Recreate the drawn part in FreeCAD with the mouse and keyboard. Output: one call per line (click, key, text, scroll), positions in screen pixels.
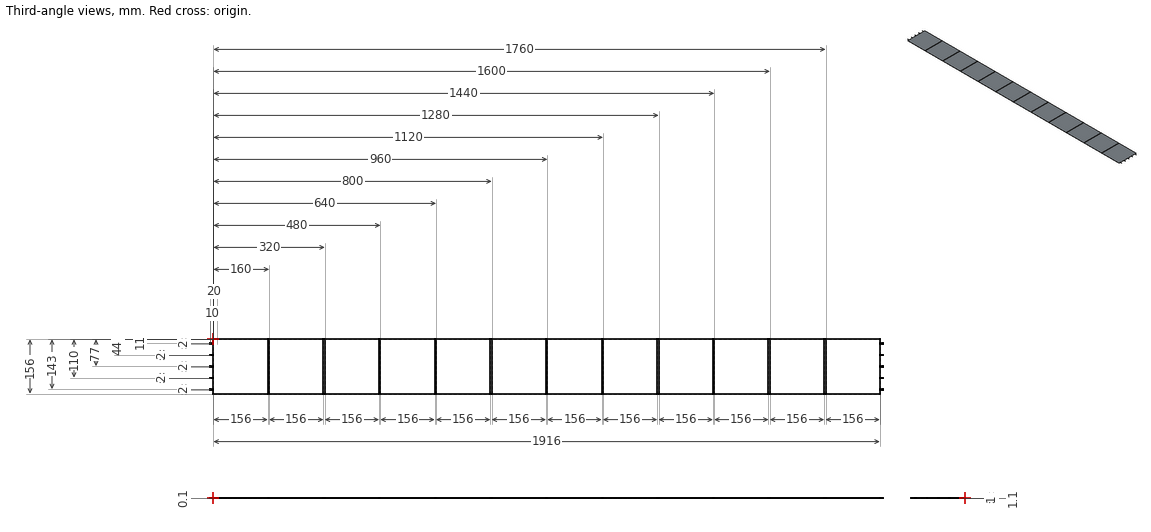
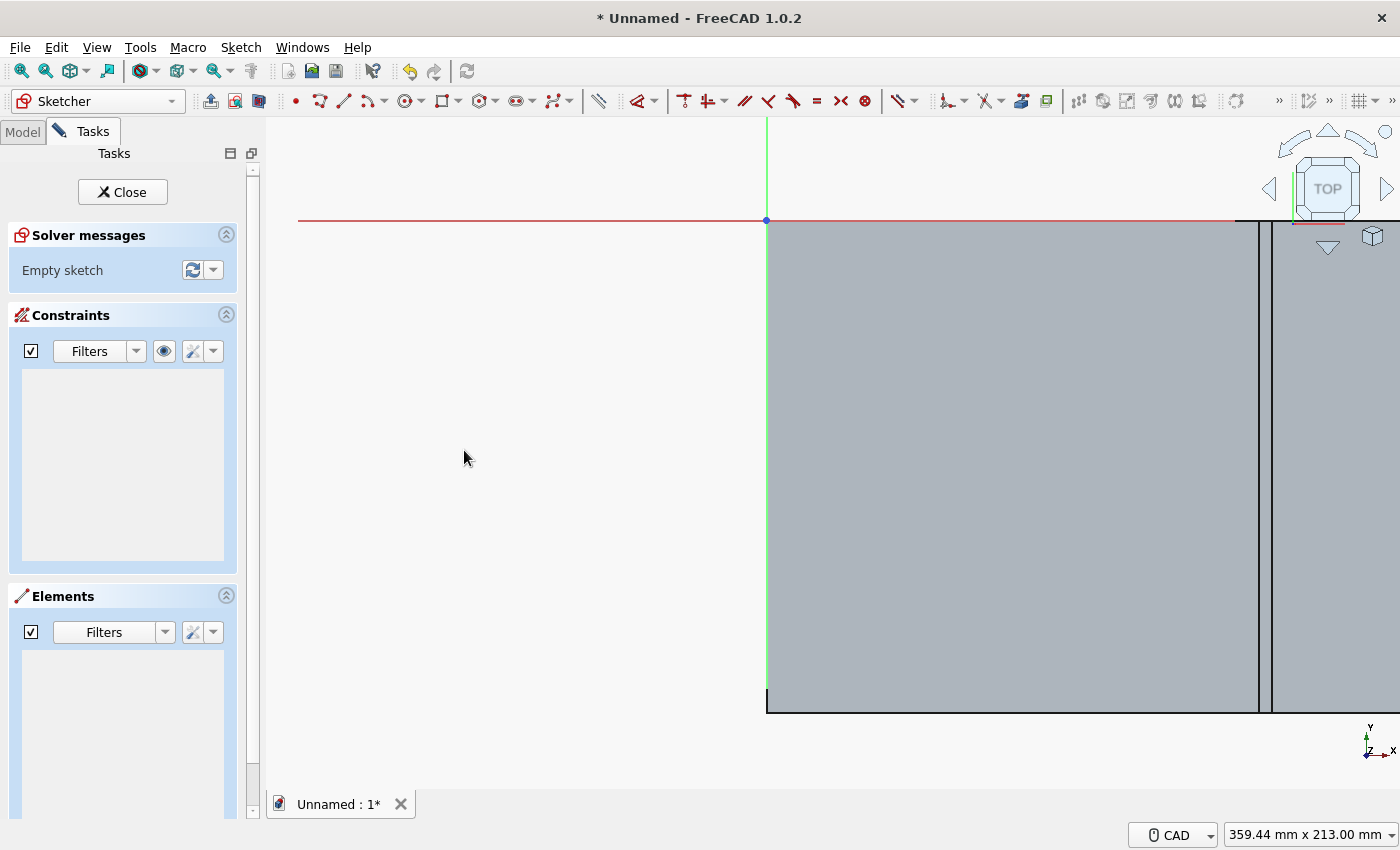
key(g)
key(r)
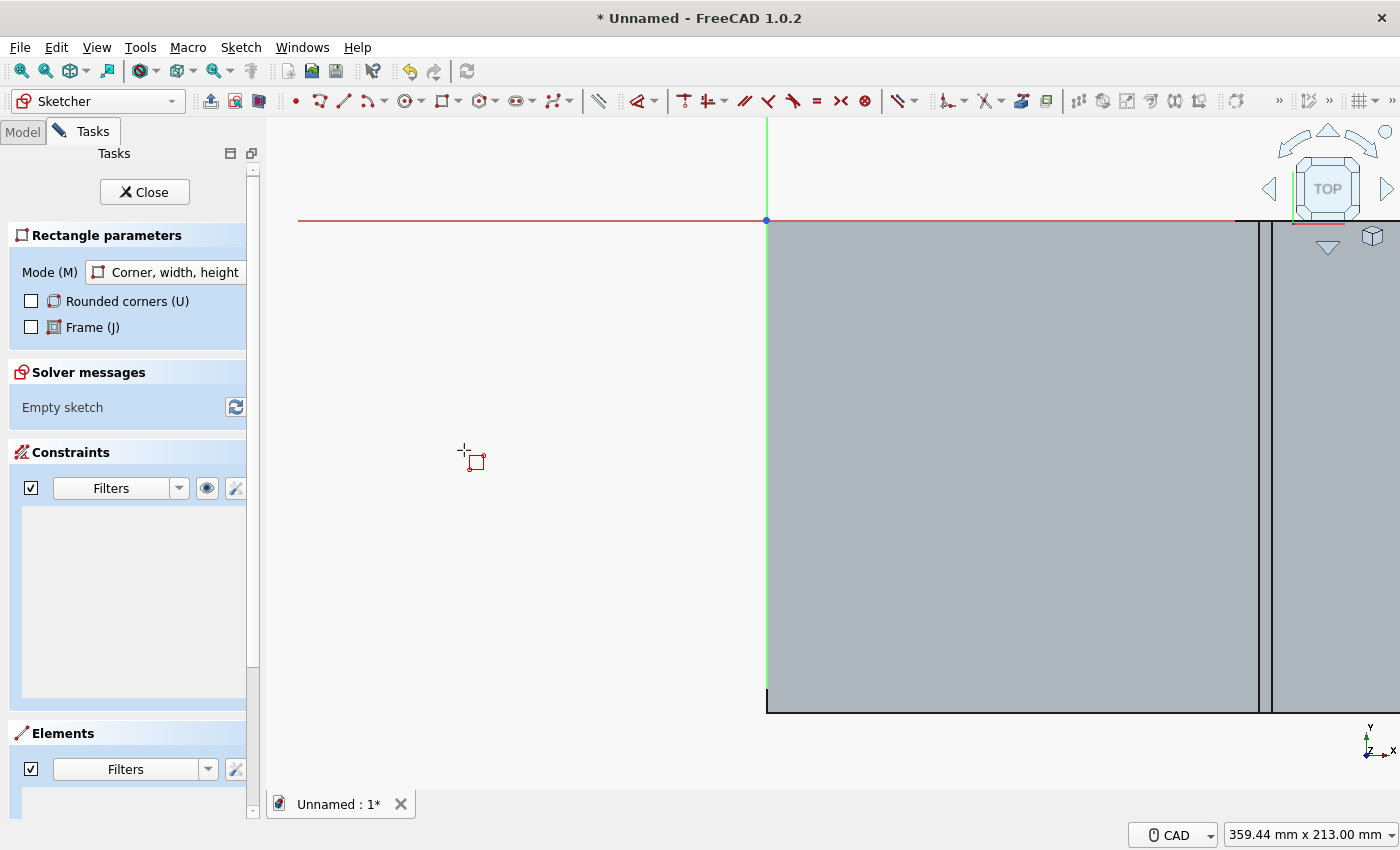
scroll(735, 255, up, 5)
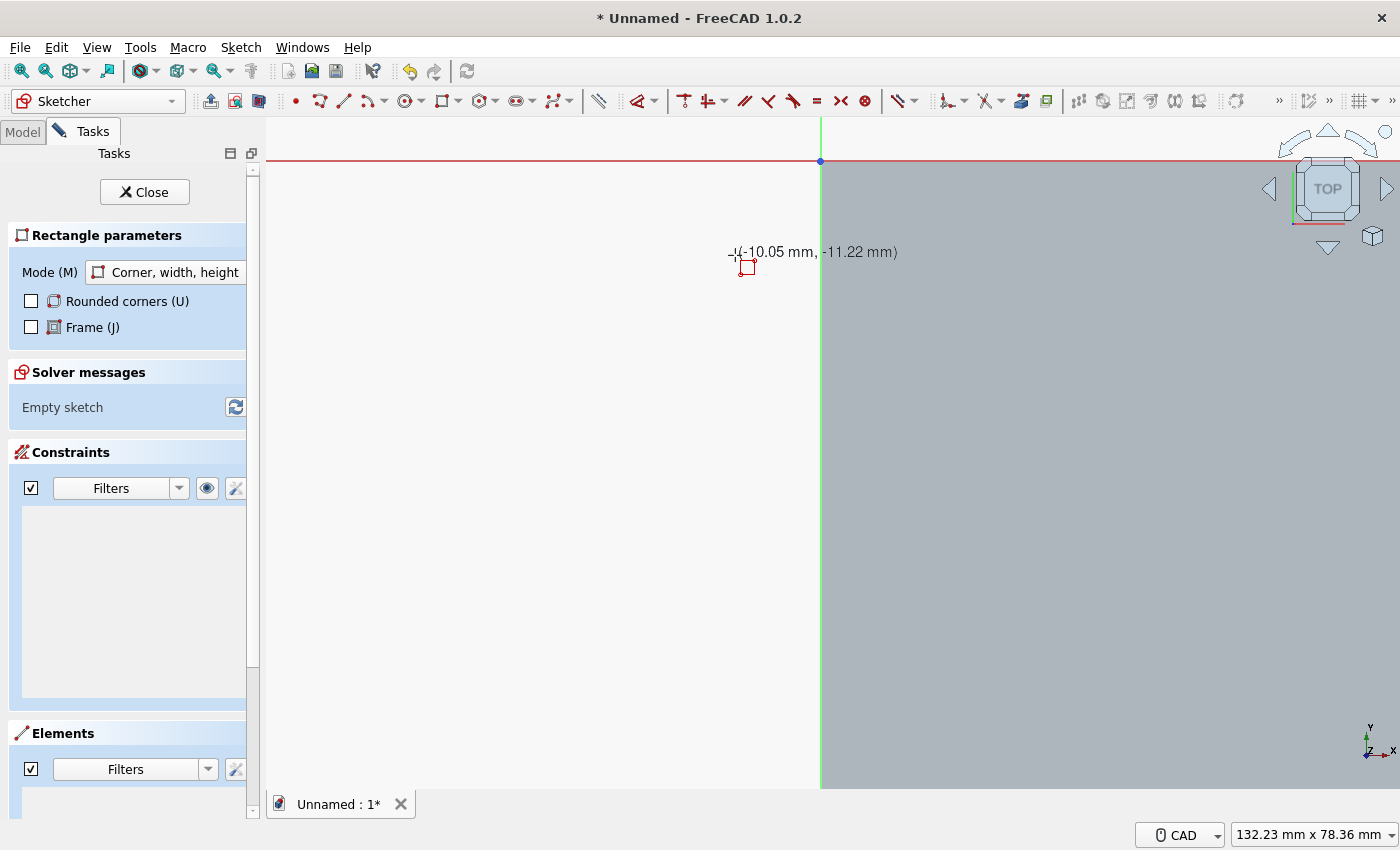
click(735, 255)
click(906, 273)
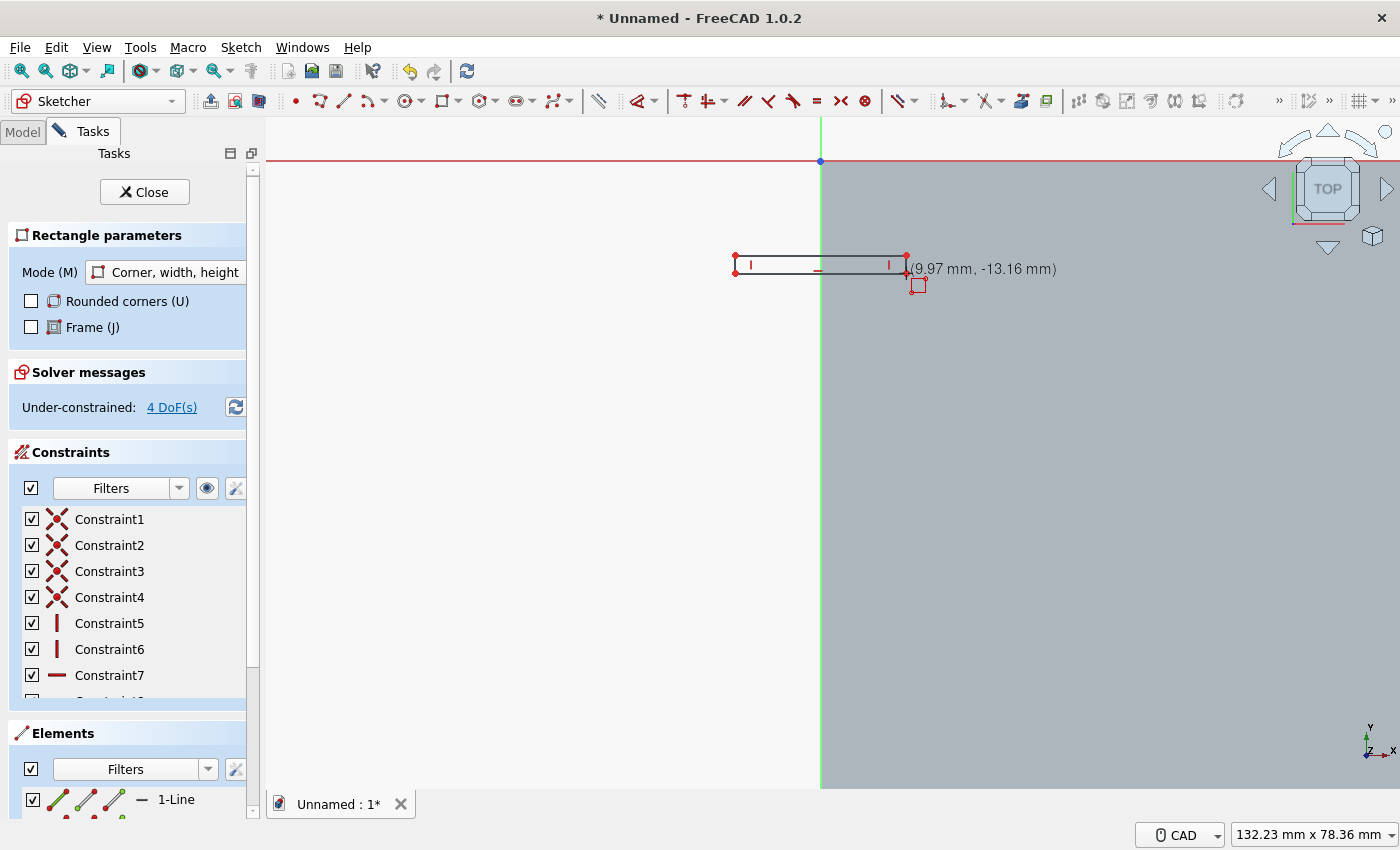
click(735, 538)
click(906, 556)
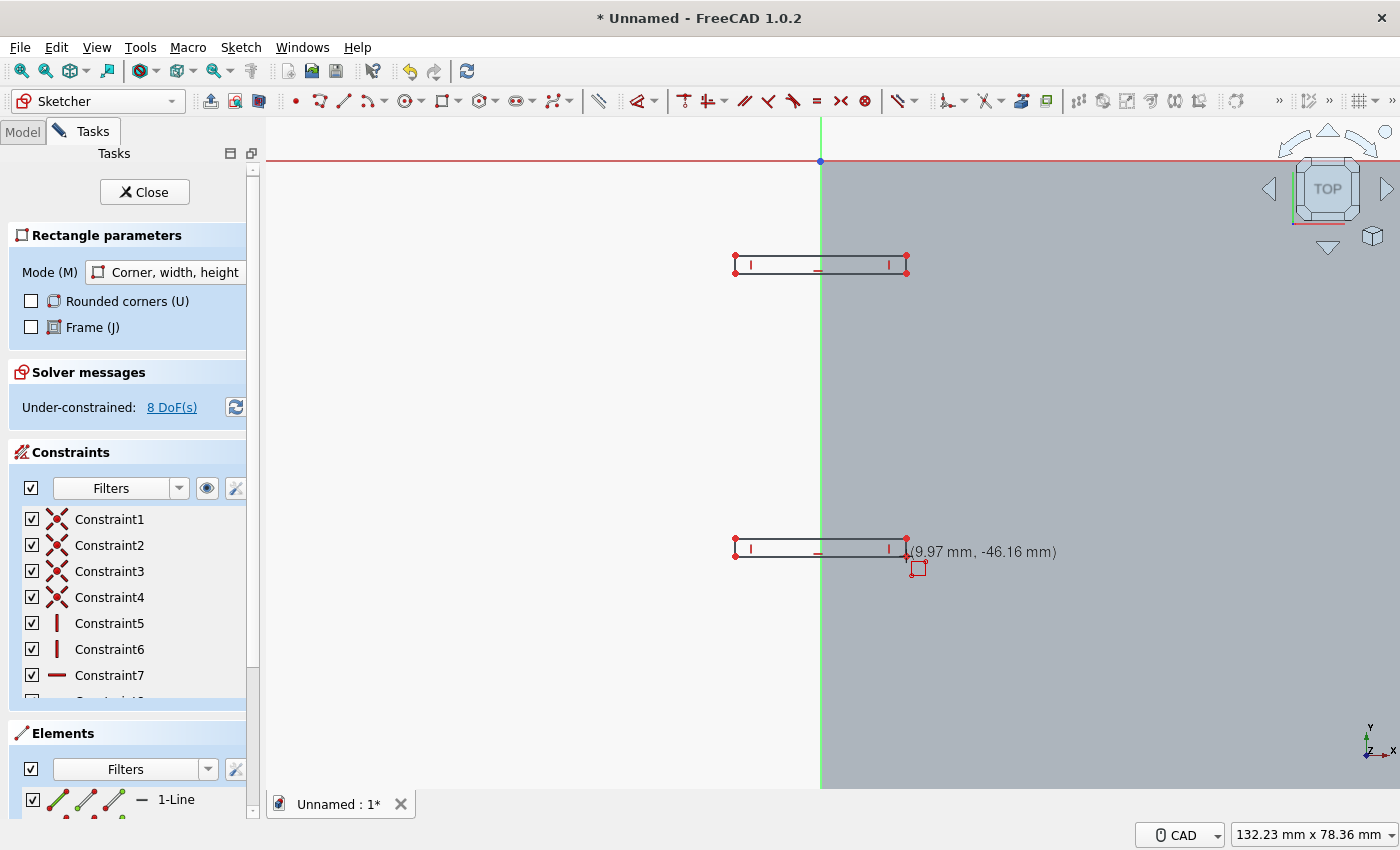
scroll(732, 261, down, 5)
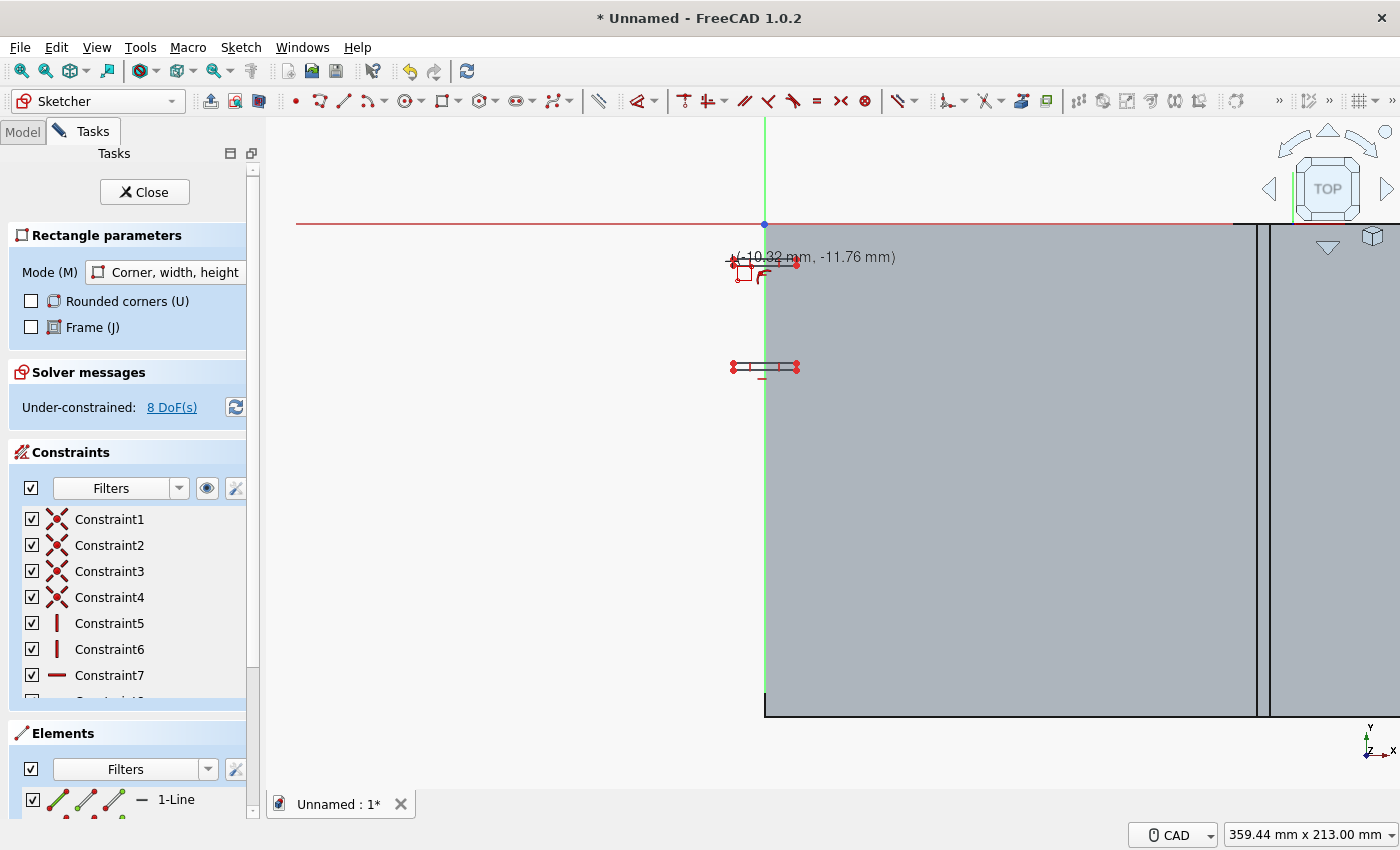
scroll(733, 467, up, 5)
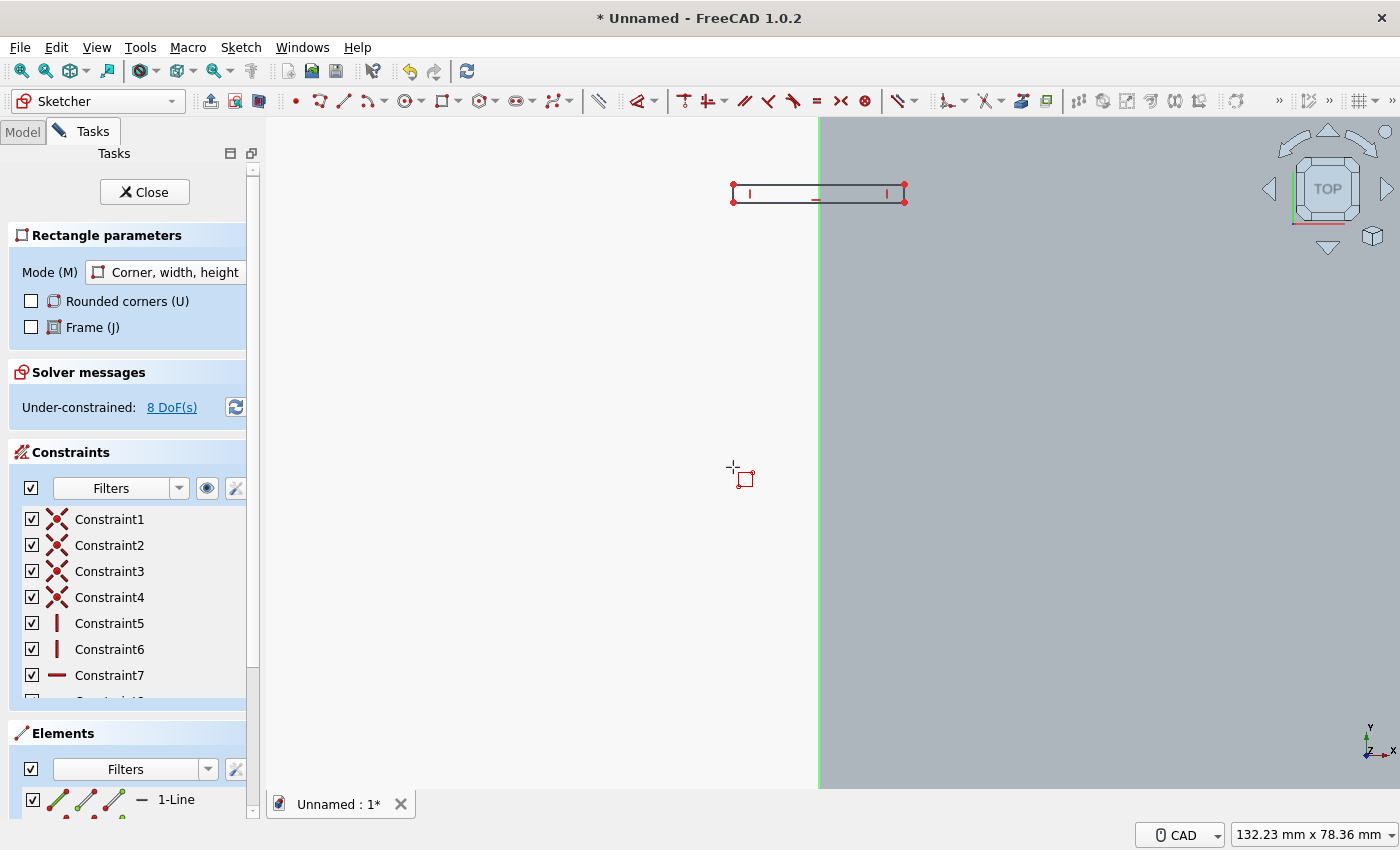
click(733, 467)
click(905, 484)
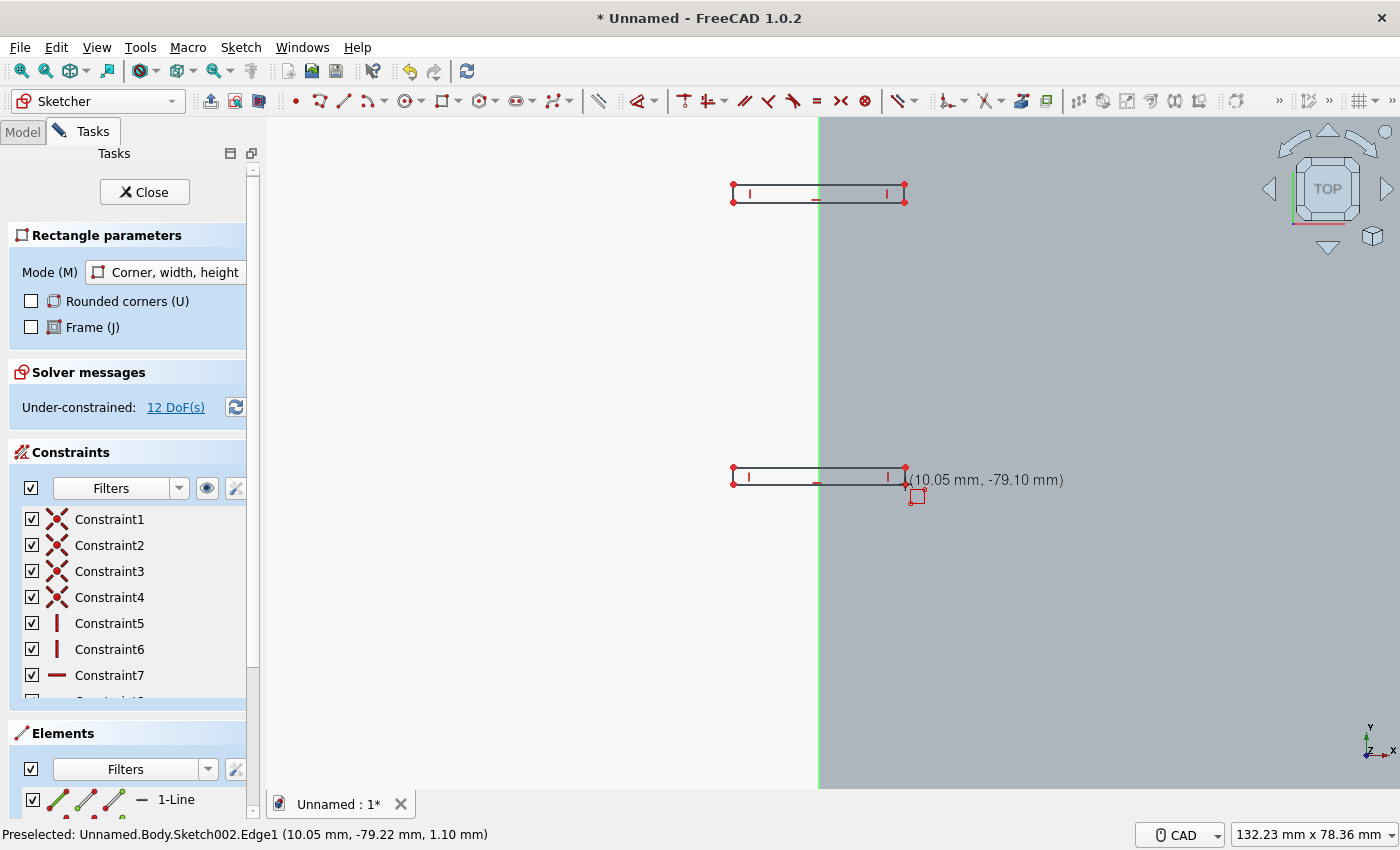
click(733, 750)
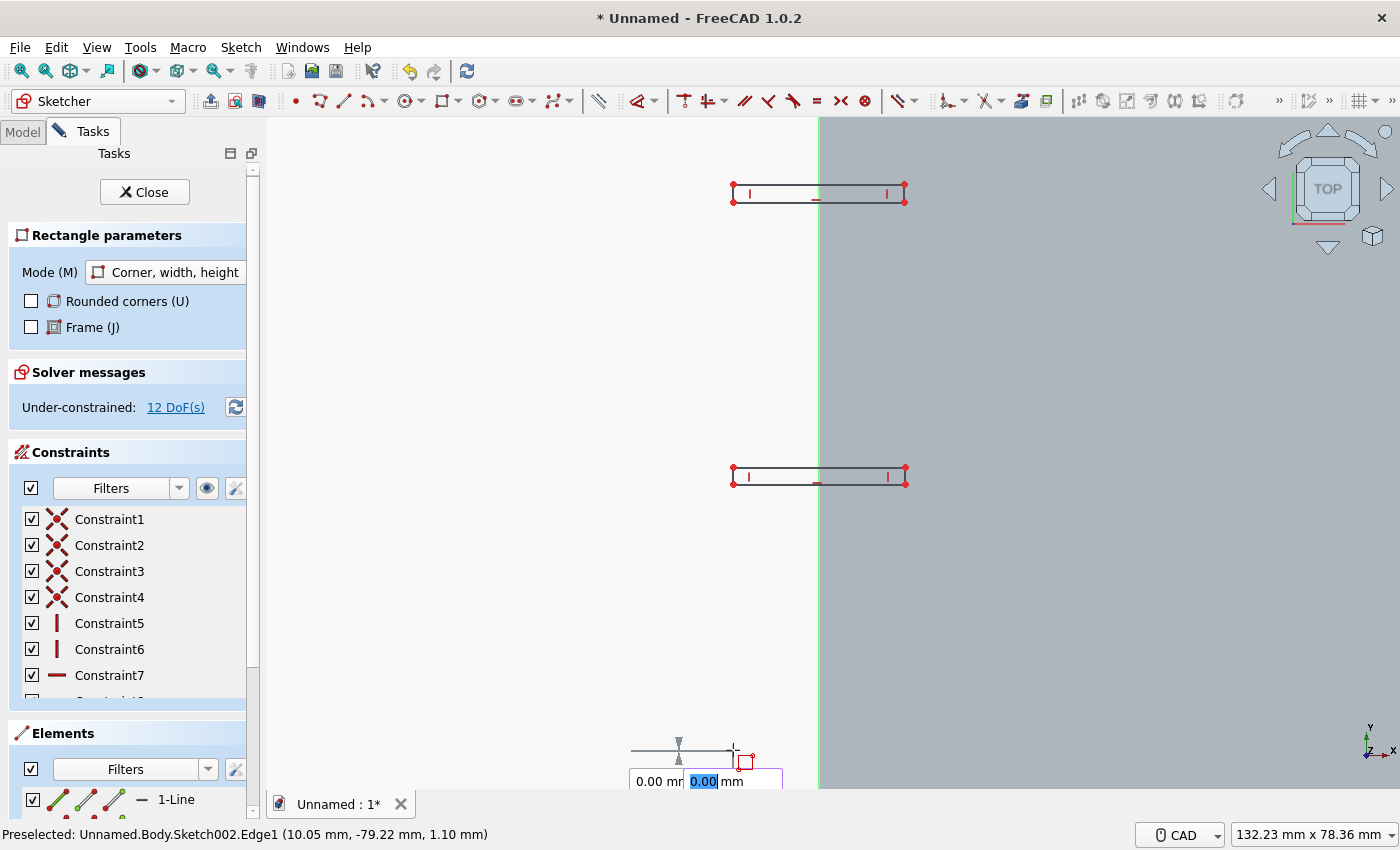
scroll(733, 467, down, 5)